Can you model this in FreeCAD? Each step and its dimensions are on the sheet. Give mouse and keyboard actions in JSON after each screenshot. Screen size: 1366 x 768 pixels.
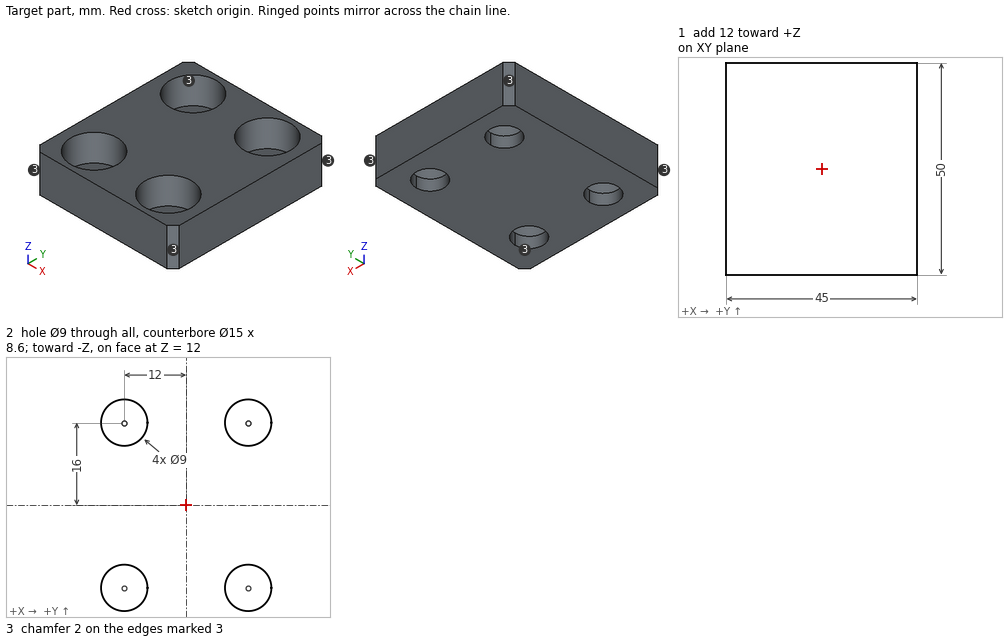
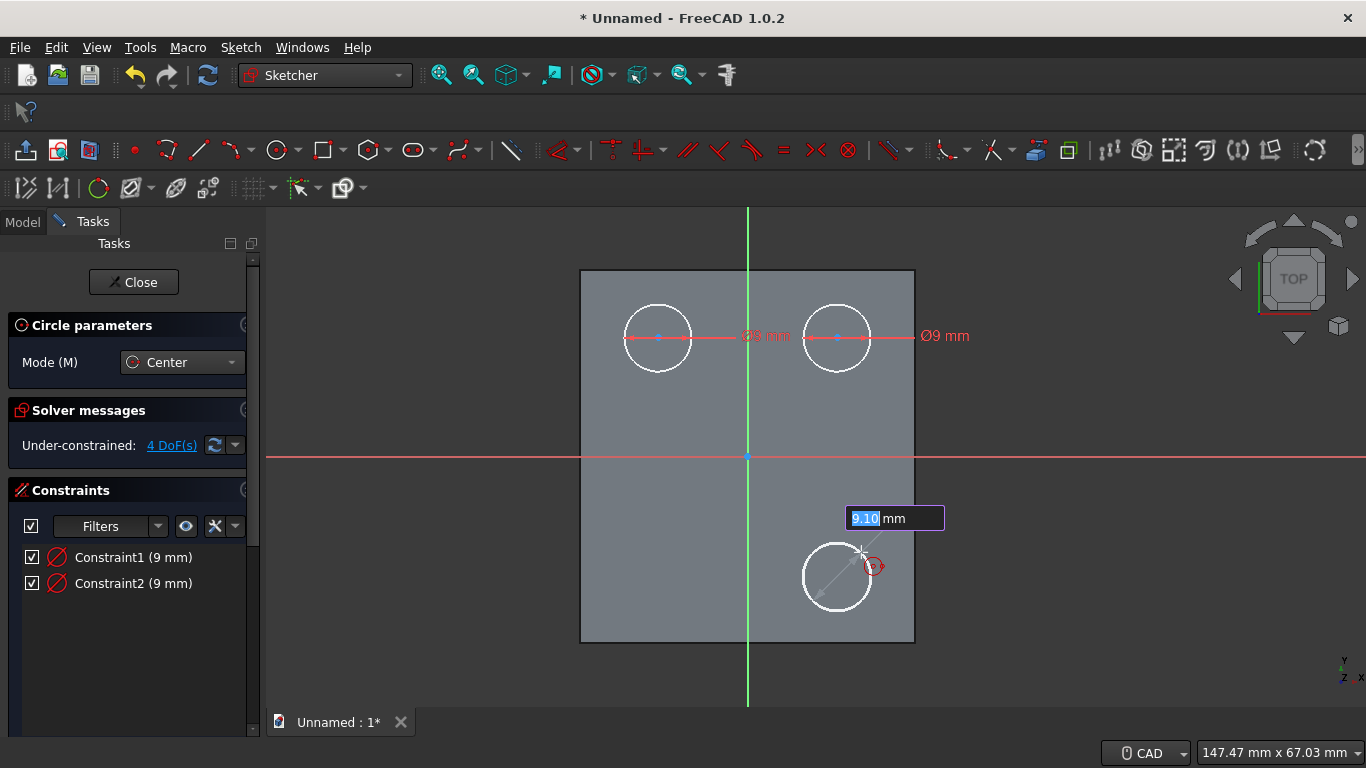
{"action": "type", "text": "9"}
{"action": "key", "text": "Return"}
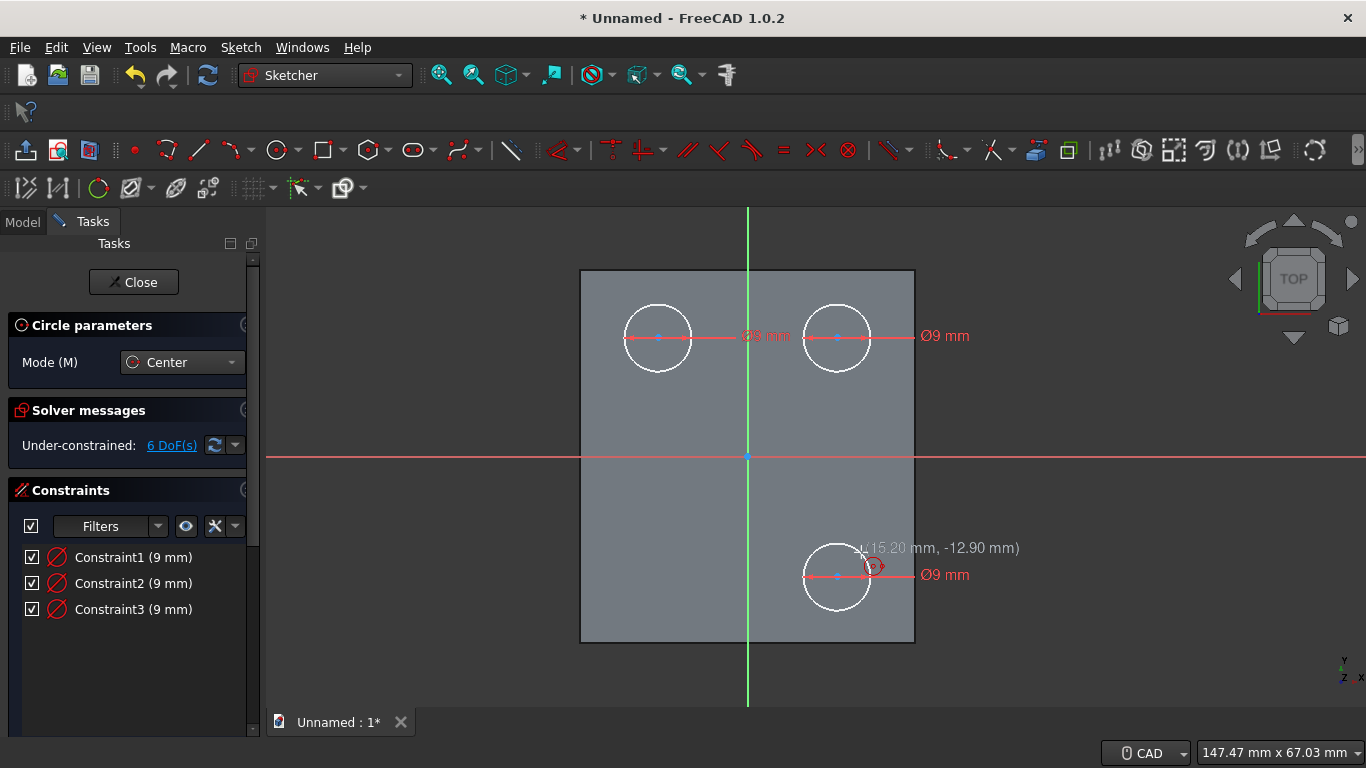
{"action": "left_click", "coordinate": [658, 576]}
{"action": "mouse_move", "coordinate": [682, 552]}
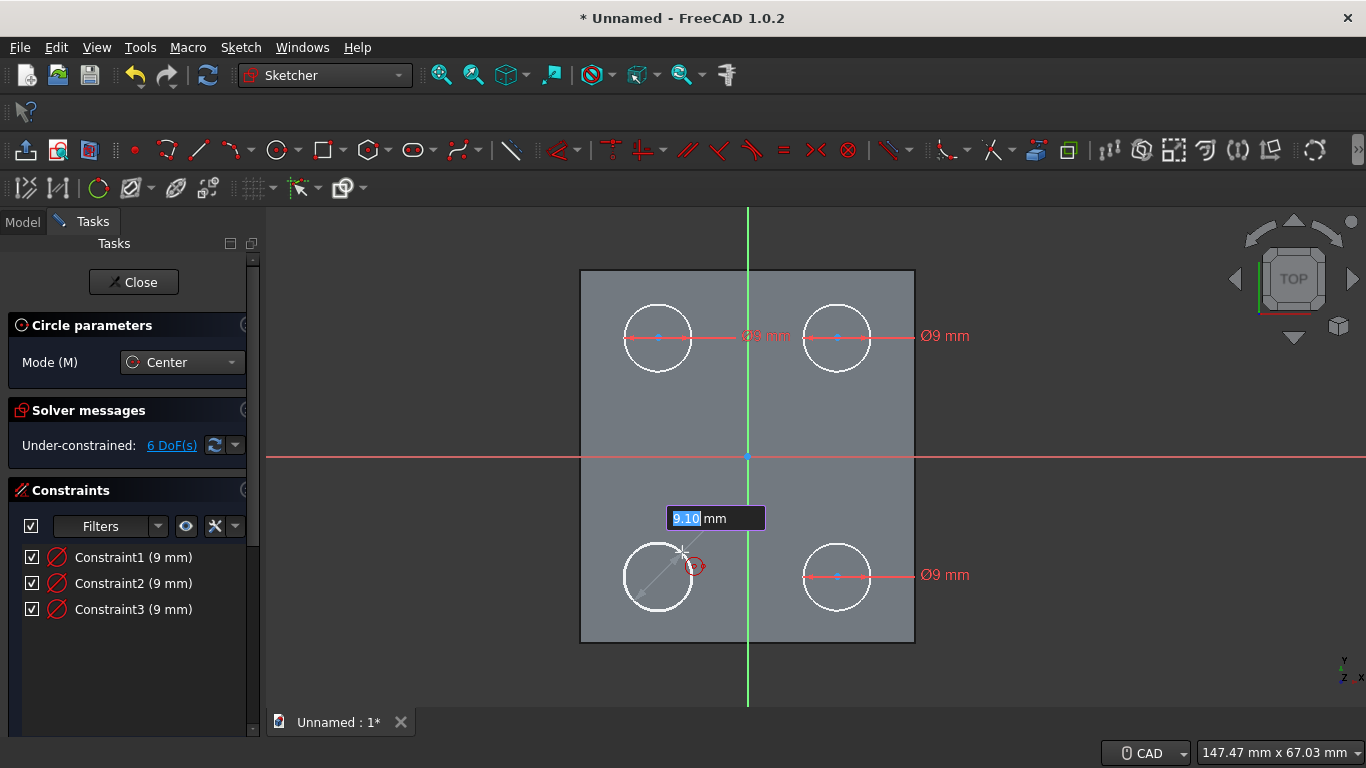
{"action": "type", "text": "9"}
{"action": "key", "text": "Return"}
{"action": "key", "text": "Escape"}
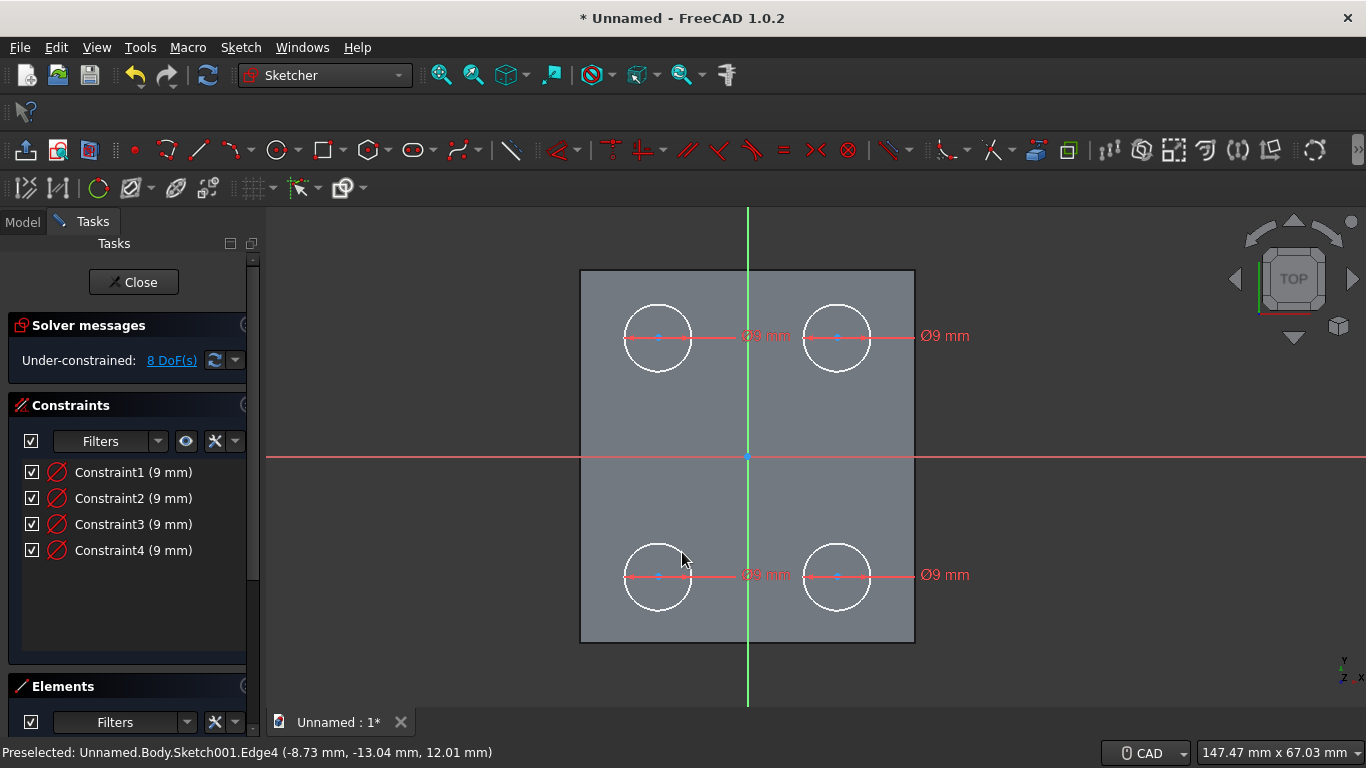
{"action": "left_click", "coordinate": [658, 338]}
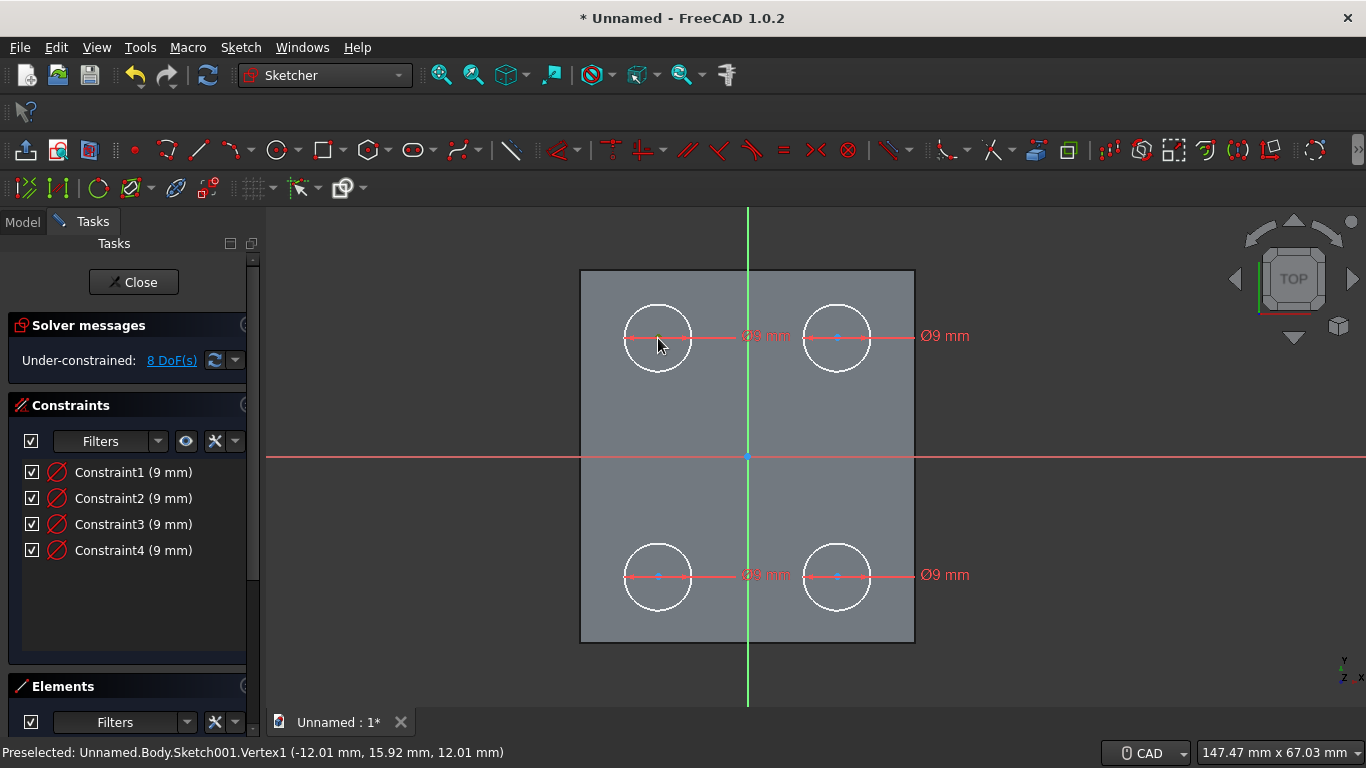
{"action": "left_click", "coordinate": [837, 338]}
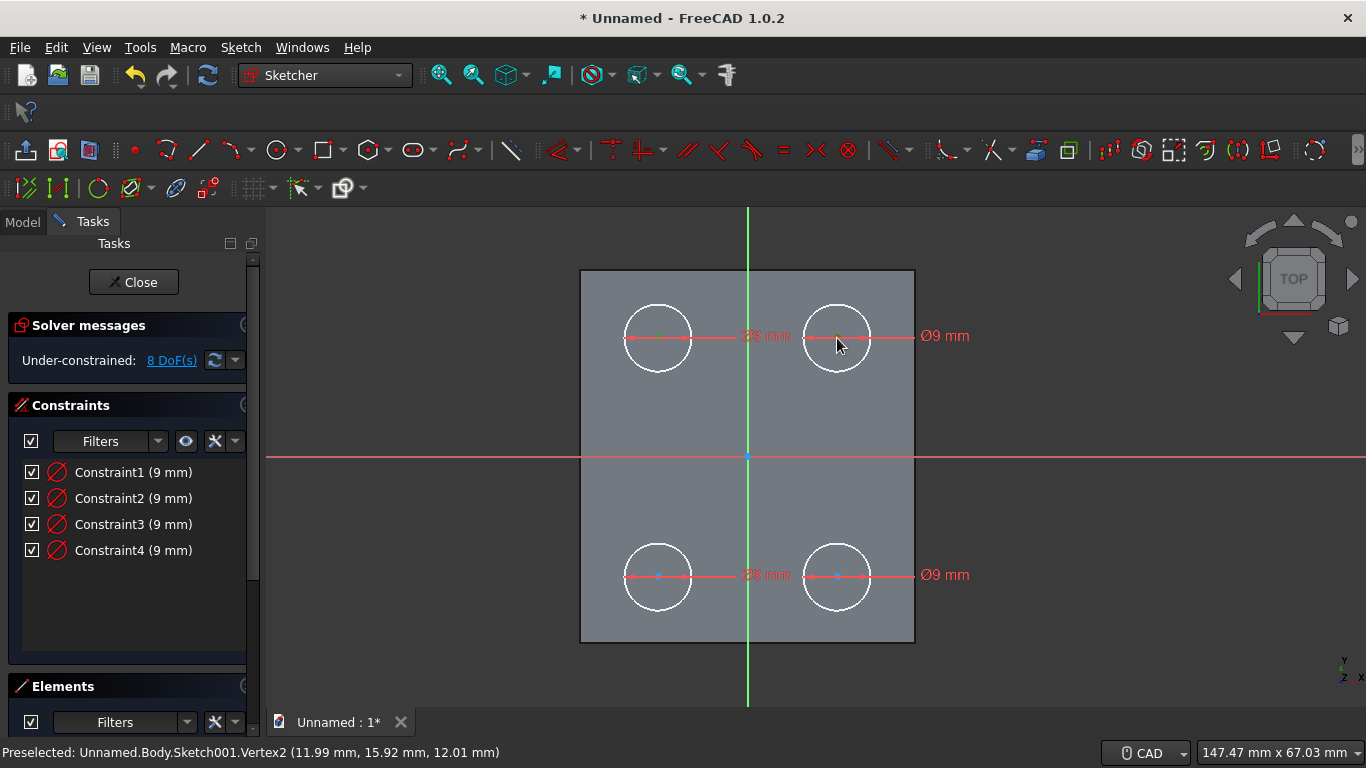
{"action": "left_click", "coordinate": [748, 647]}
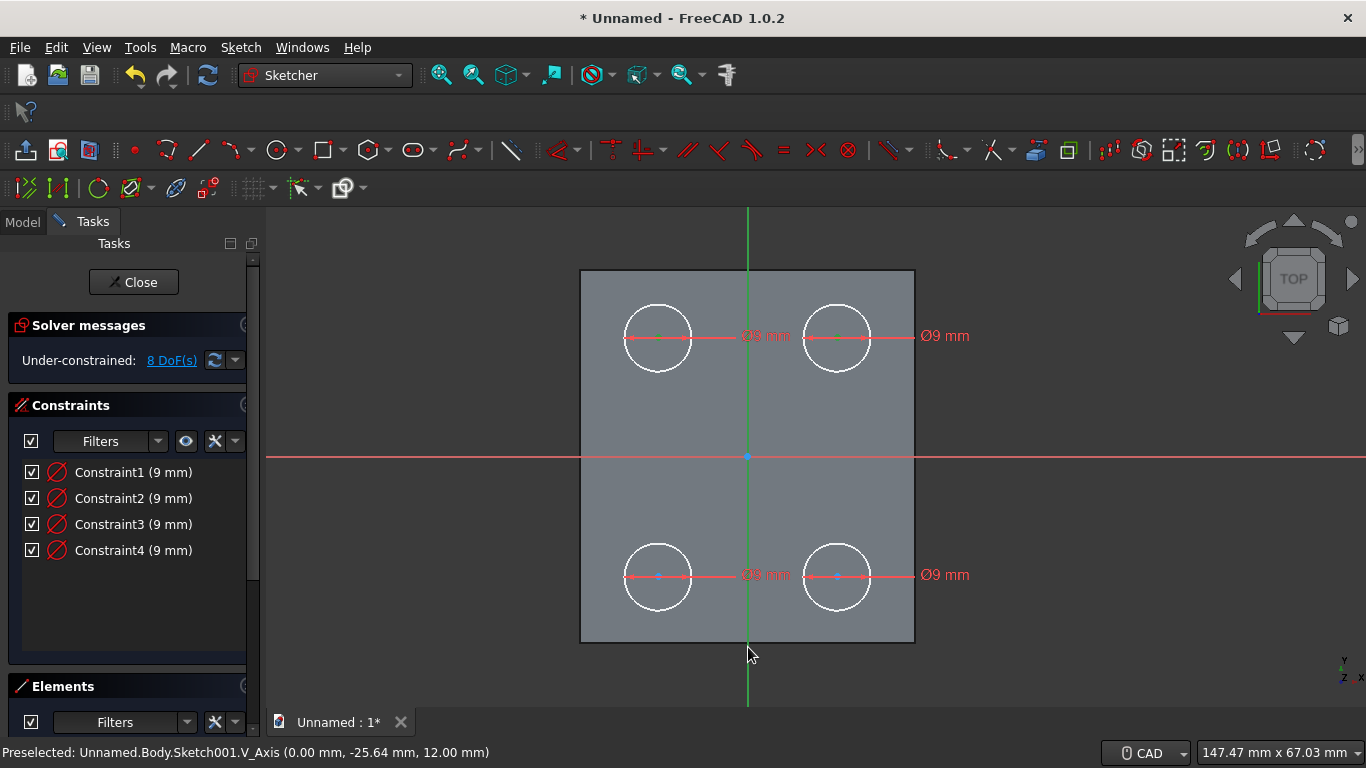
{"action": "left_click", "coordinate": [816, 150]}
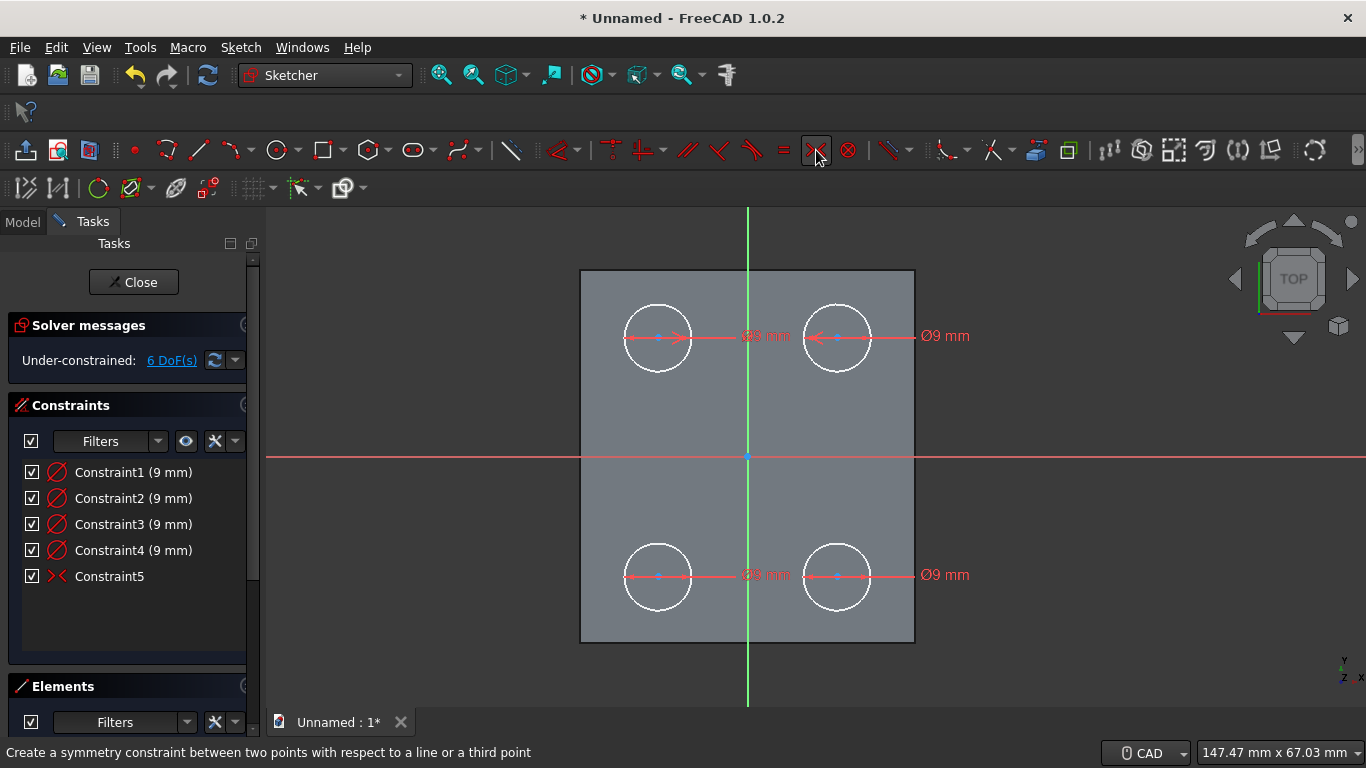
{"action": "left_click", "coordinate": [837, 338]}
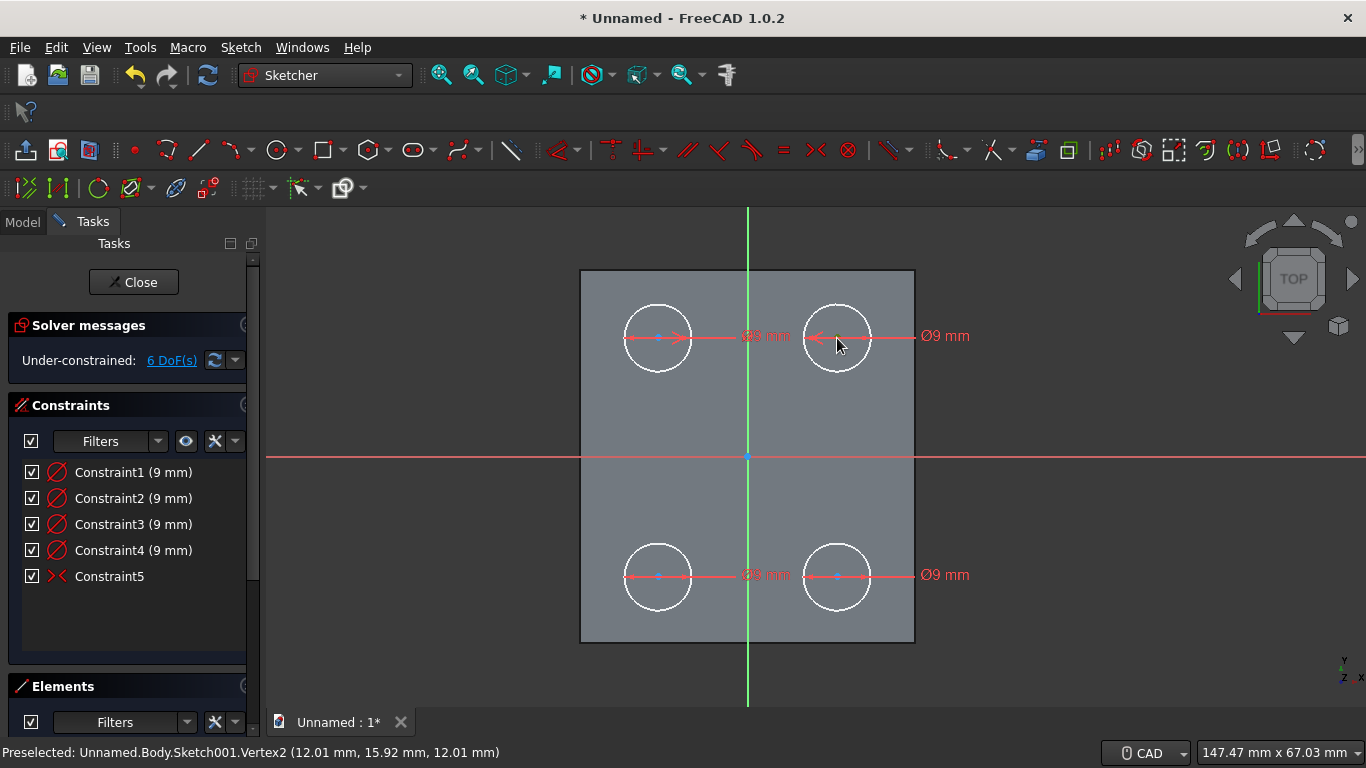
{"action": "left_click", "coordinate": [837, 577]}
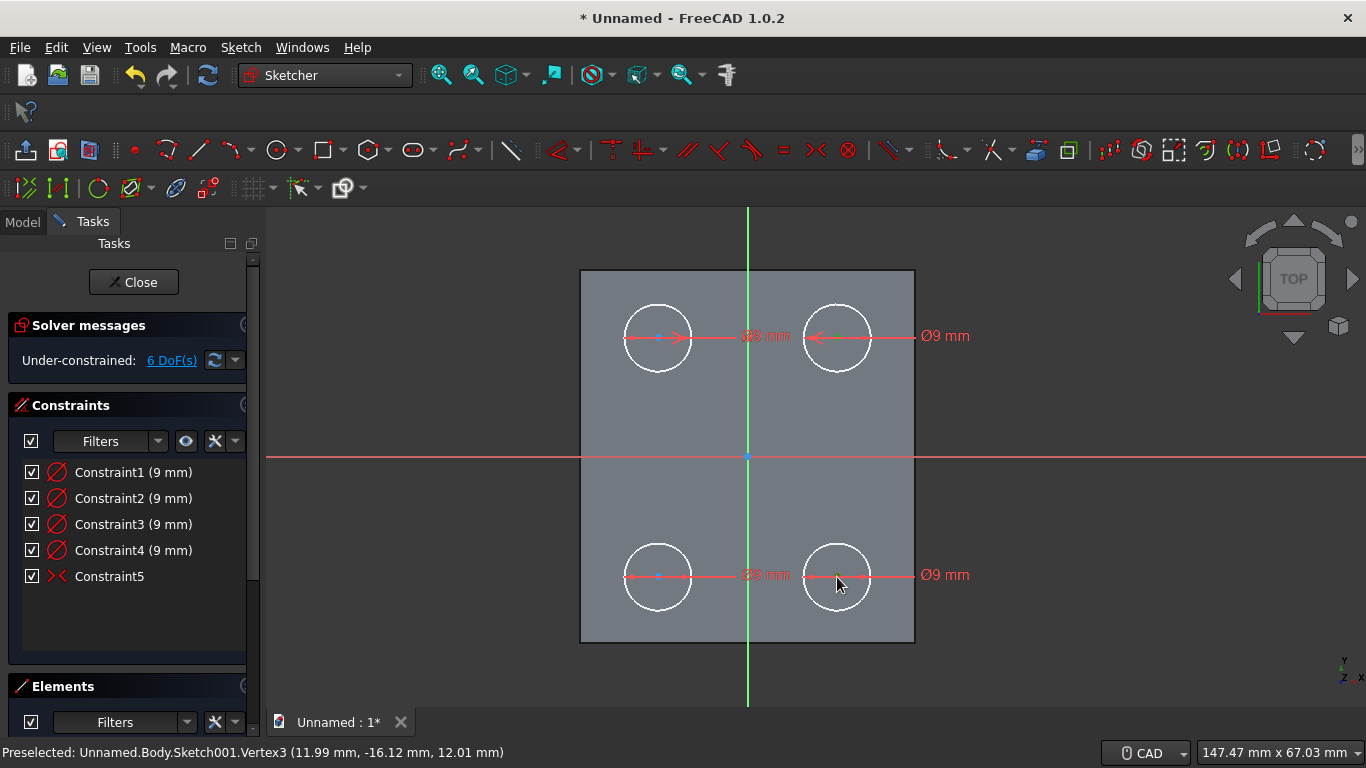
{"action": "left_click", "coordinate": [359, 457]}